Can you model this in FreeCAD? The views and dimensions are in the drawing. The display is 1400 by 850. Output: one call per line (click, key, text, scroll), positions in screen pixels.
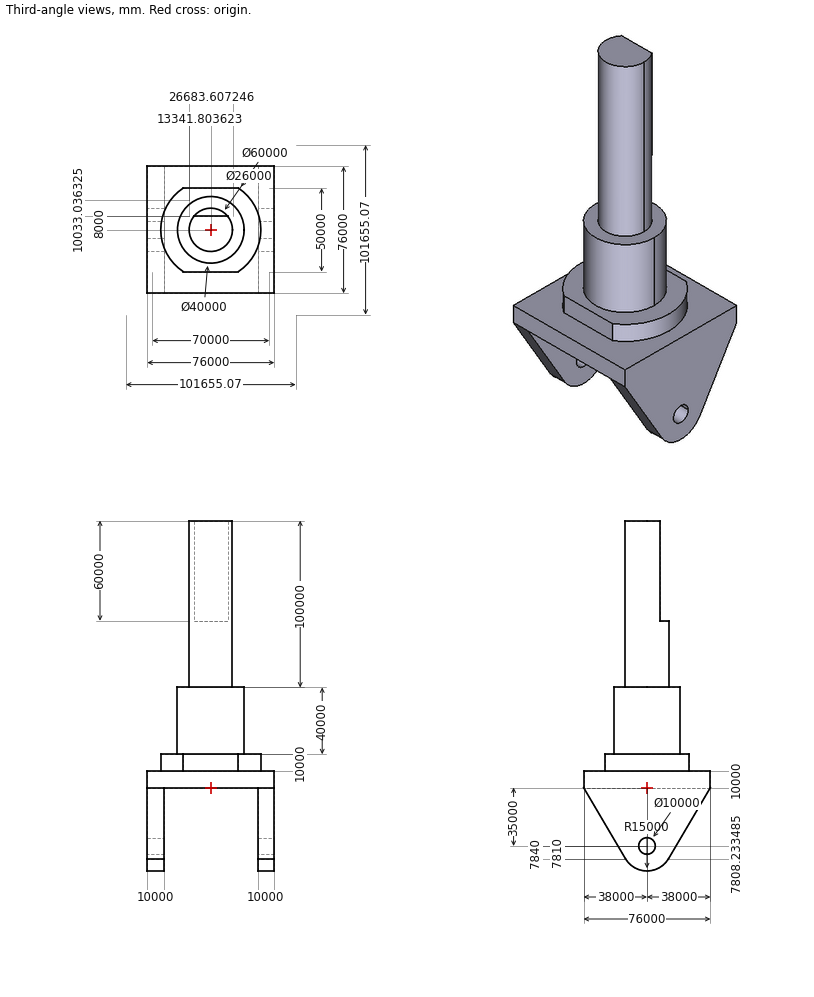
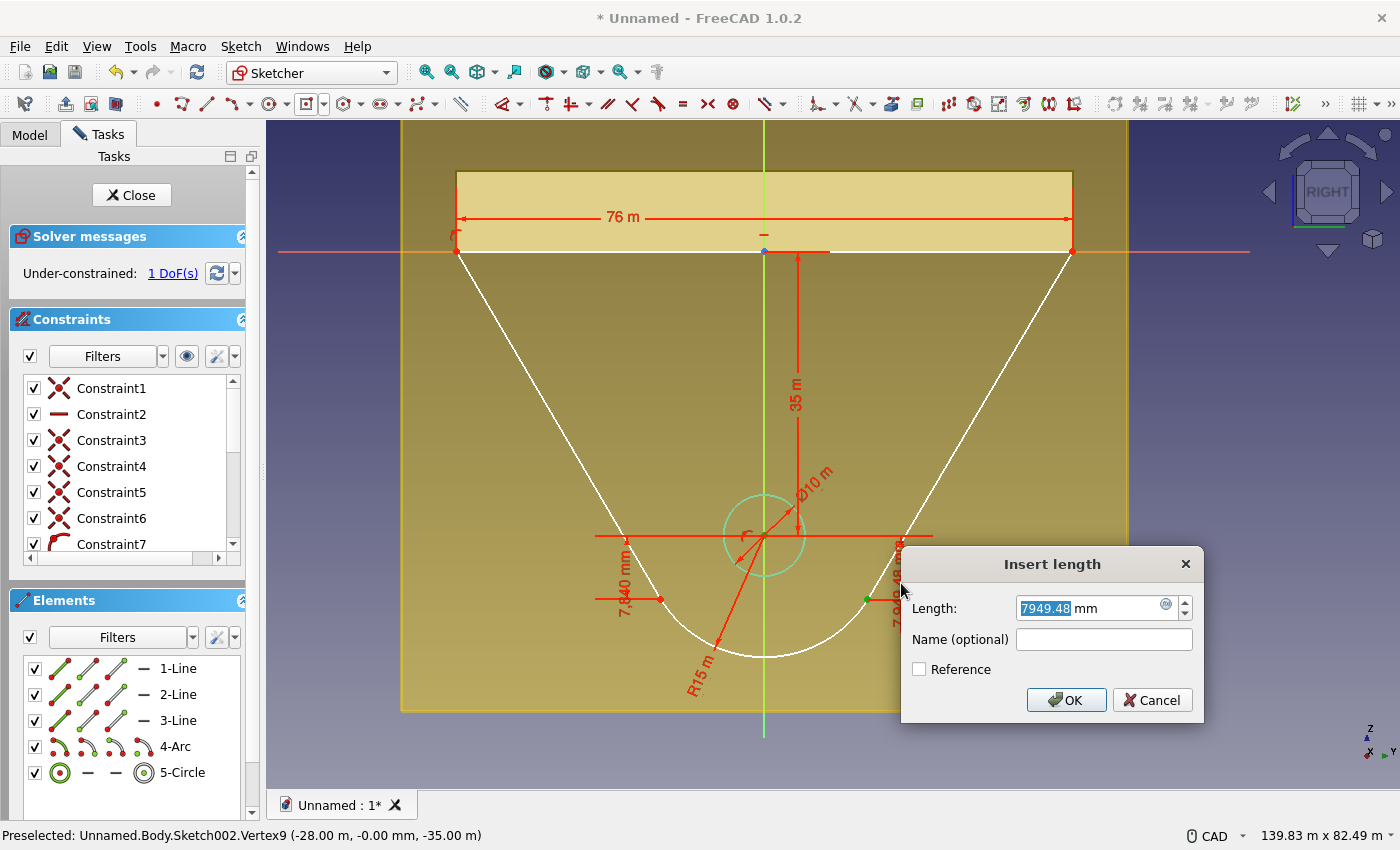
text(7840)
key(Return)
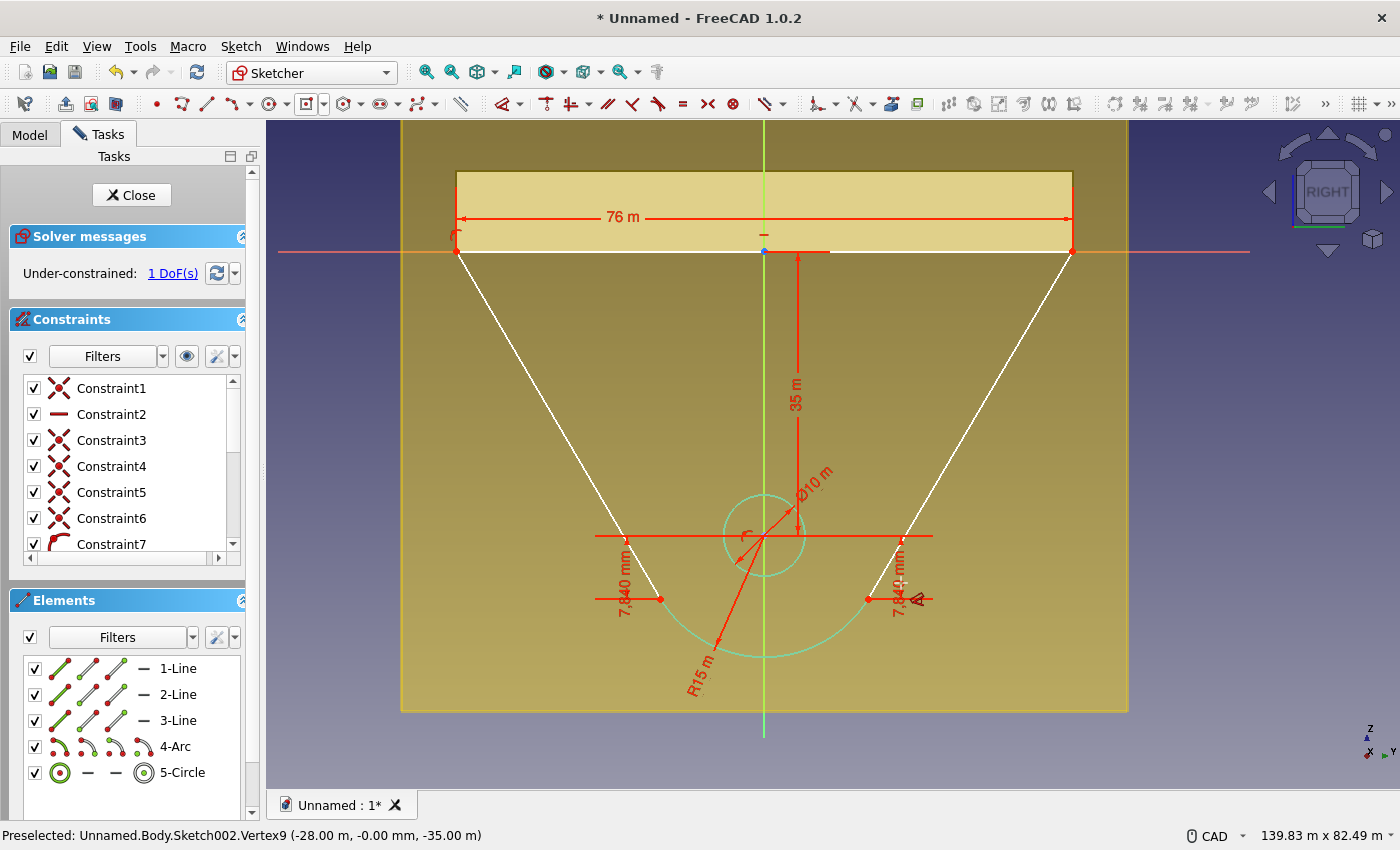
click(456, 252)
click(540, 218)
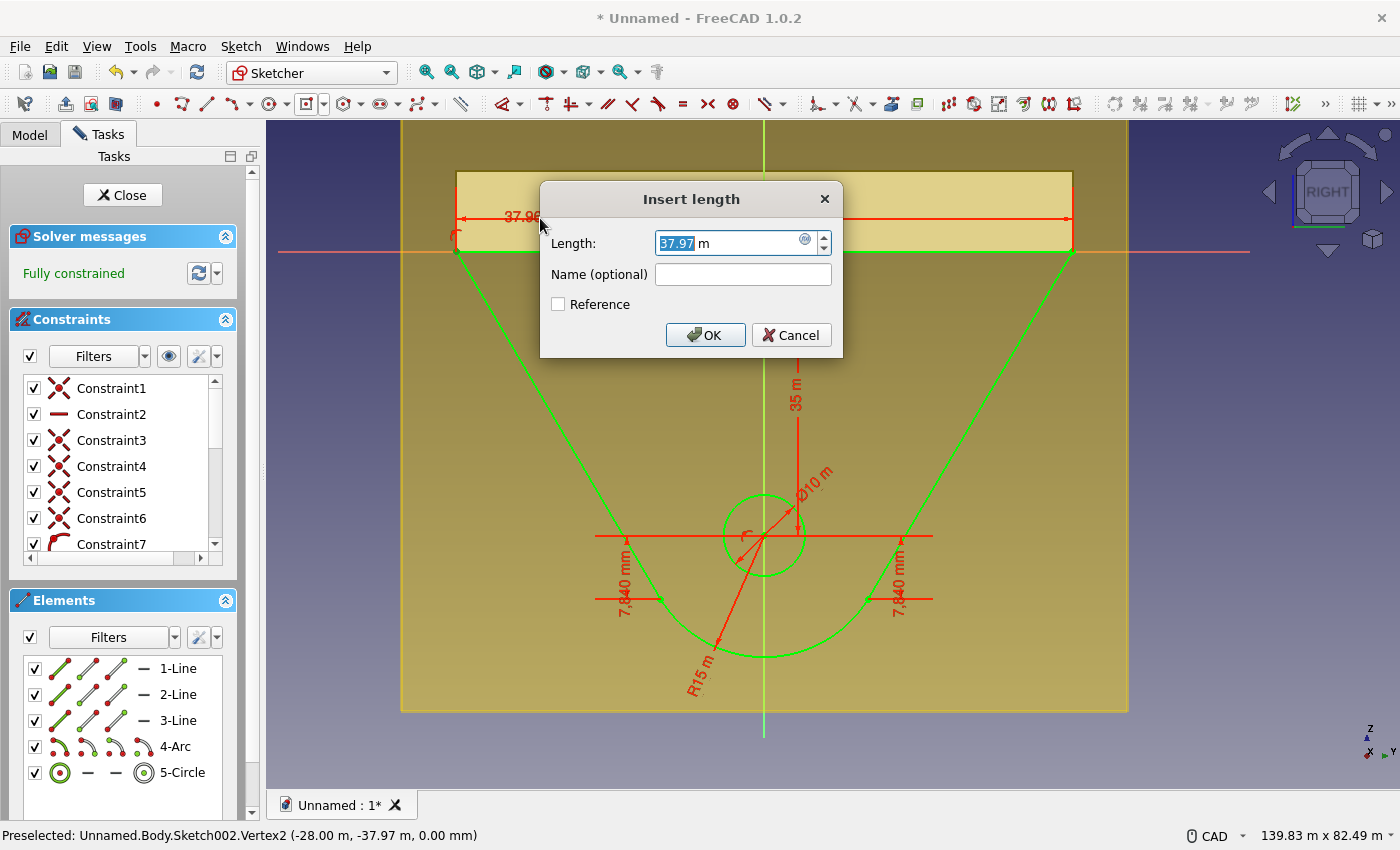
key(ctrl+a)
text(38000 mm)
key(Return)
key(Escape)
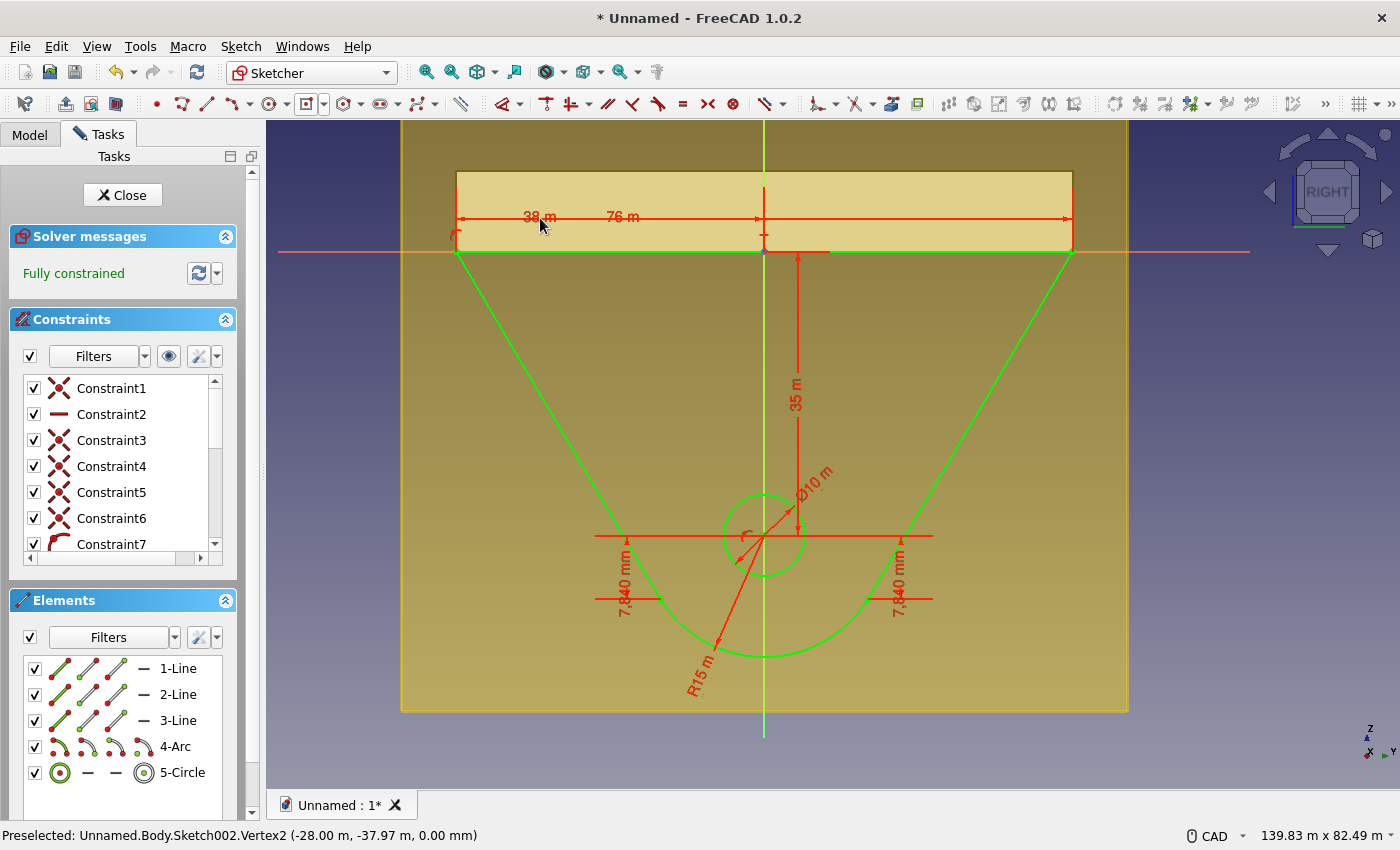
click(123, 195)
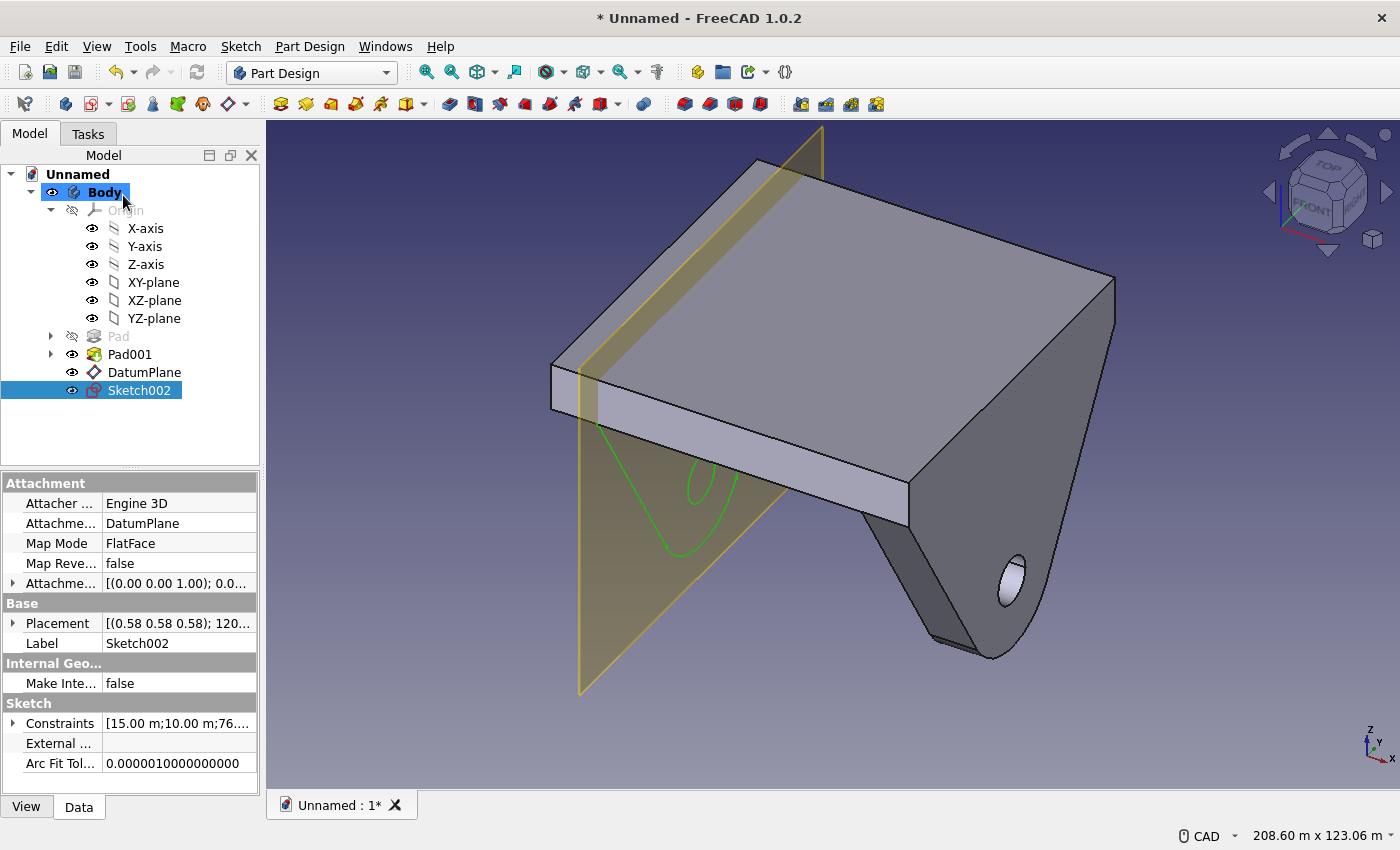
click(281, 104)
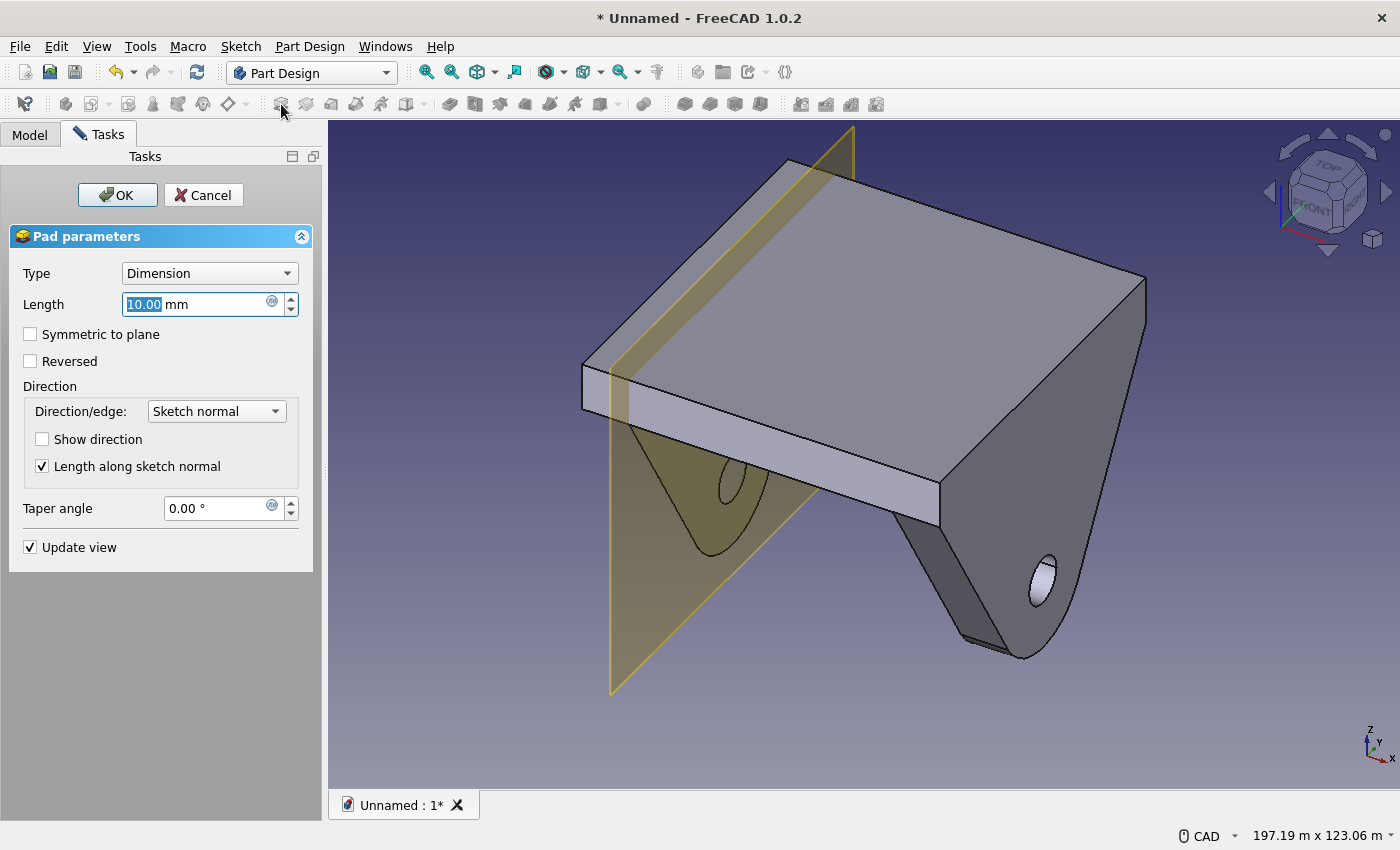
text(10000)
key(Tab)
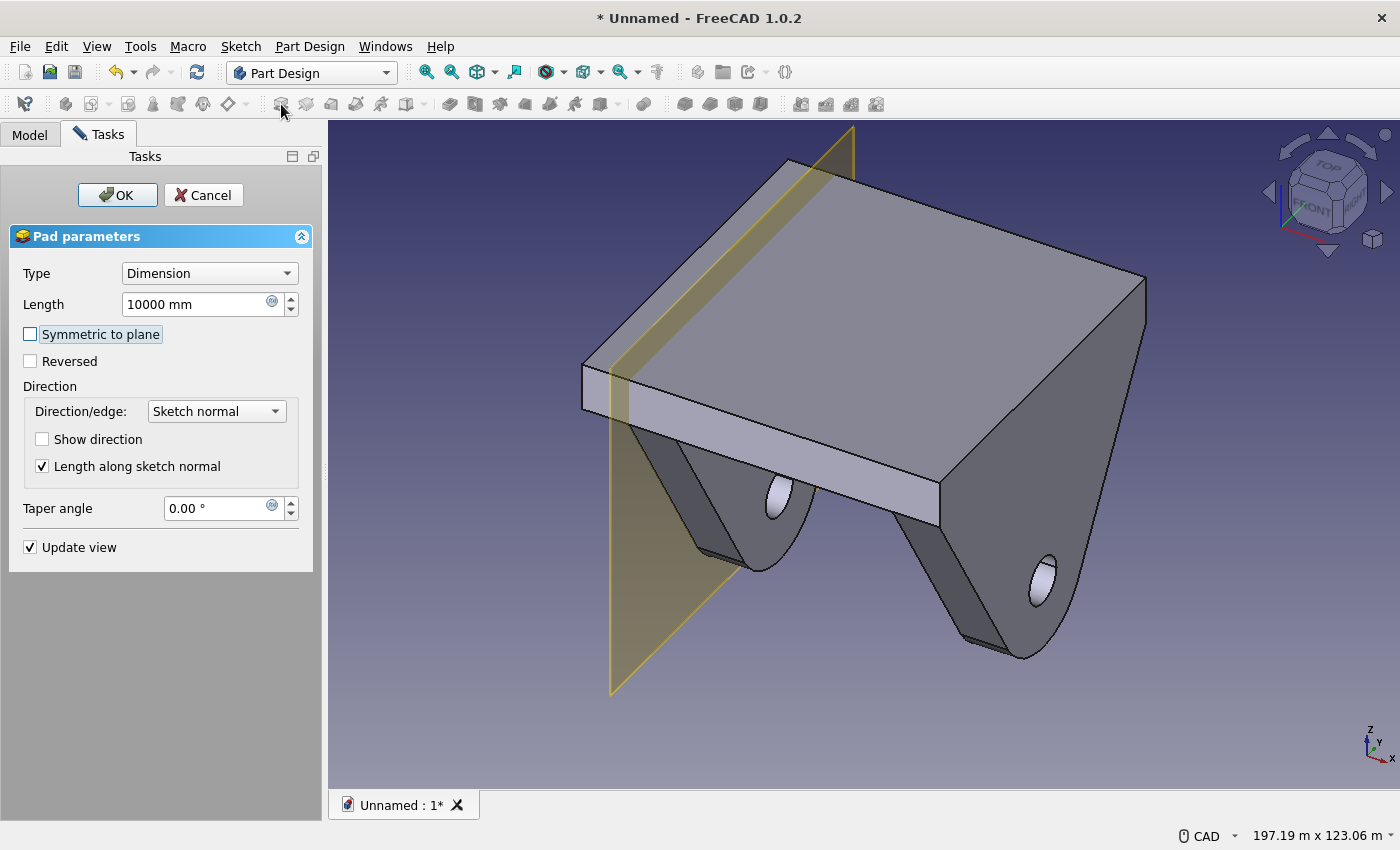
click(31, 361)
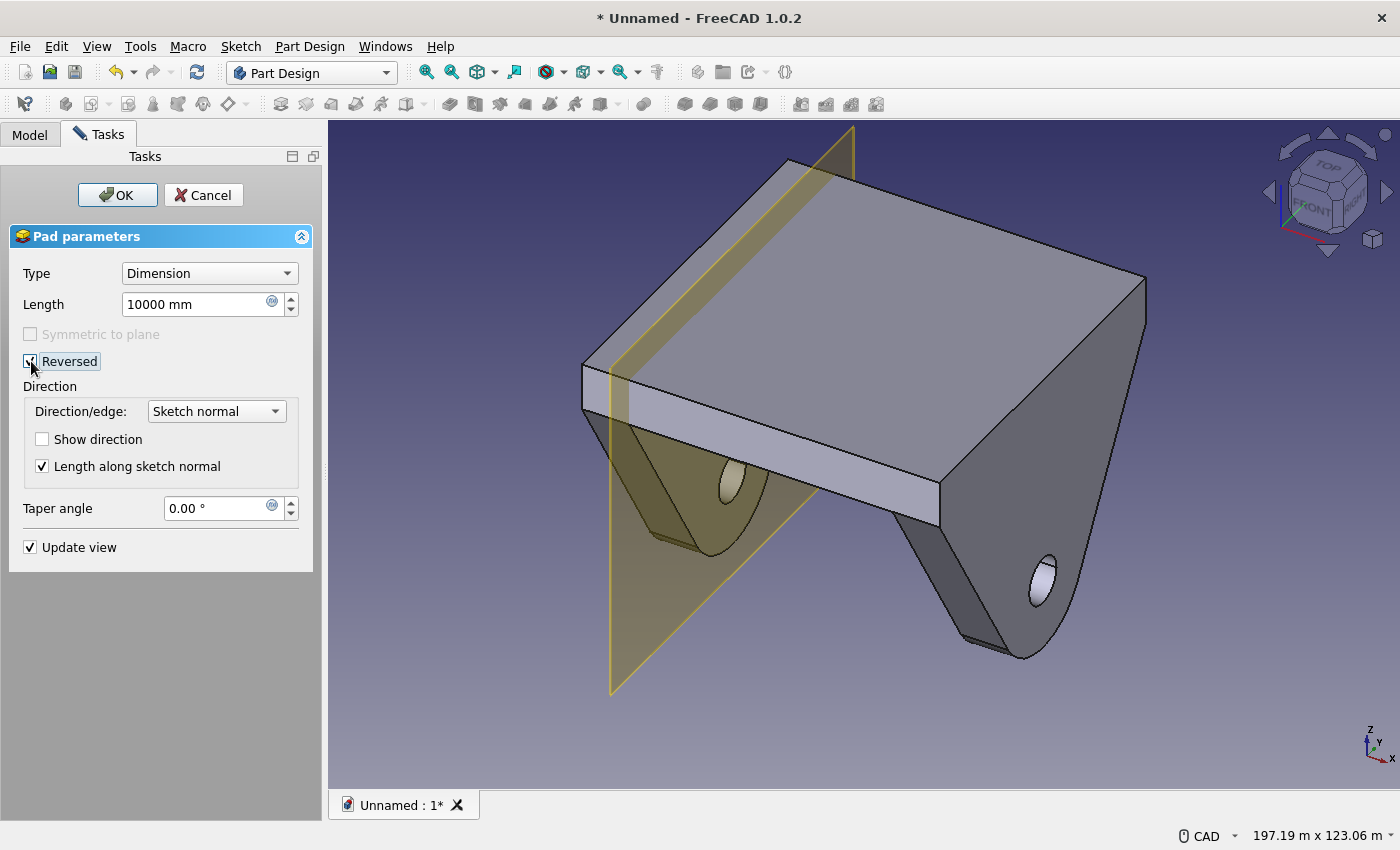
click(118, 195)